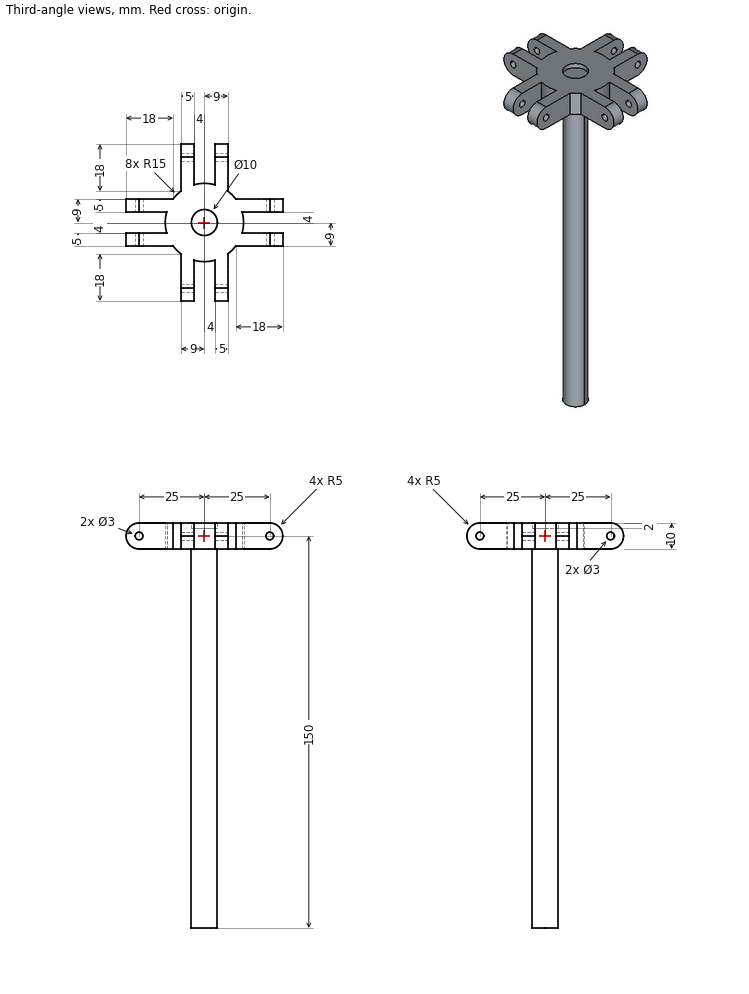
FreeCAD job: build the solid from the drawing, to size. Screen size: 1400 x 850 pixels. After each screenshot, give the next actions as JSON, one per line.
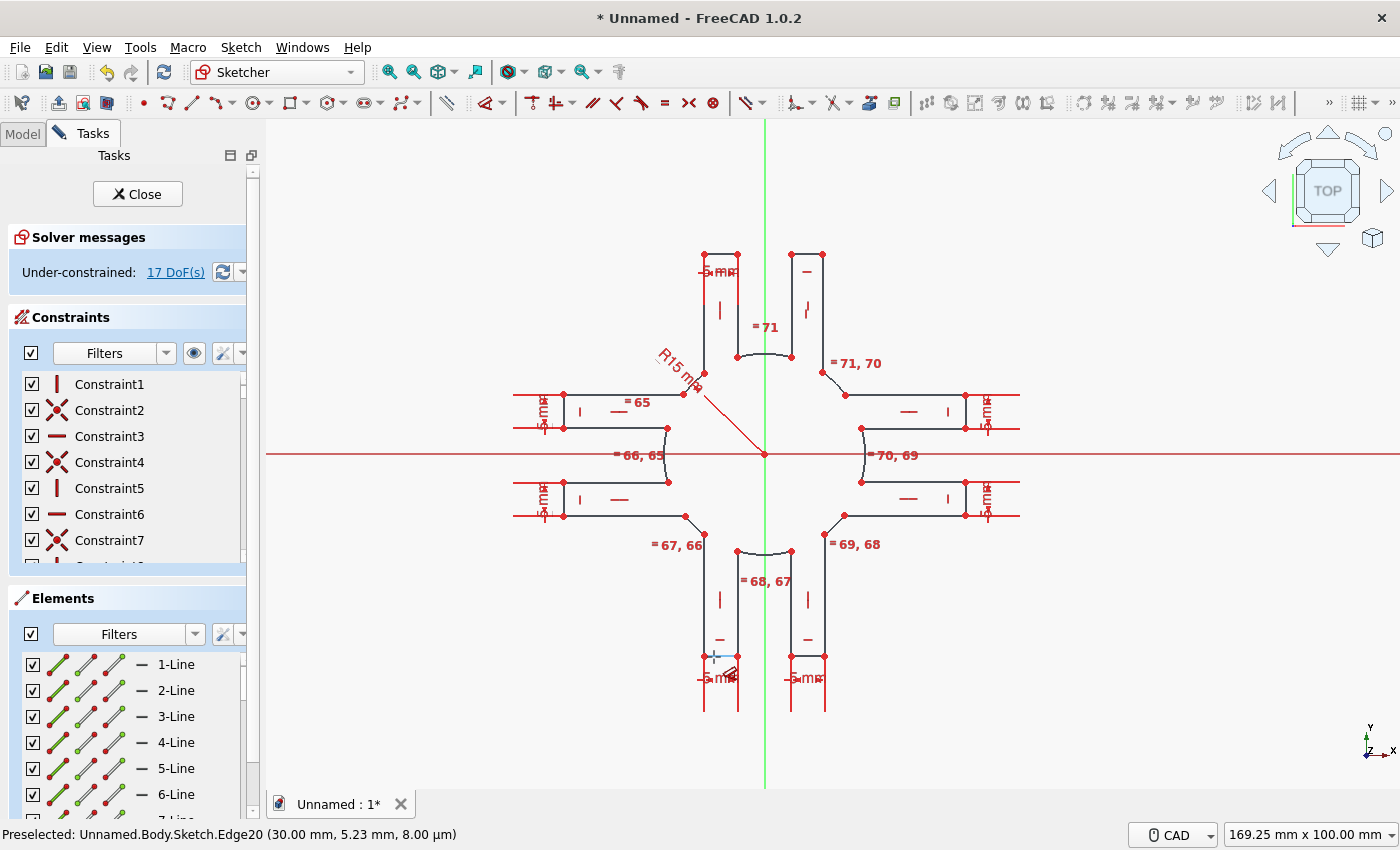
{"action": "scroll", "coordinate": [813, 254], "scroll_direction": "up", "scroll_amount": 2}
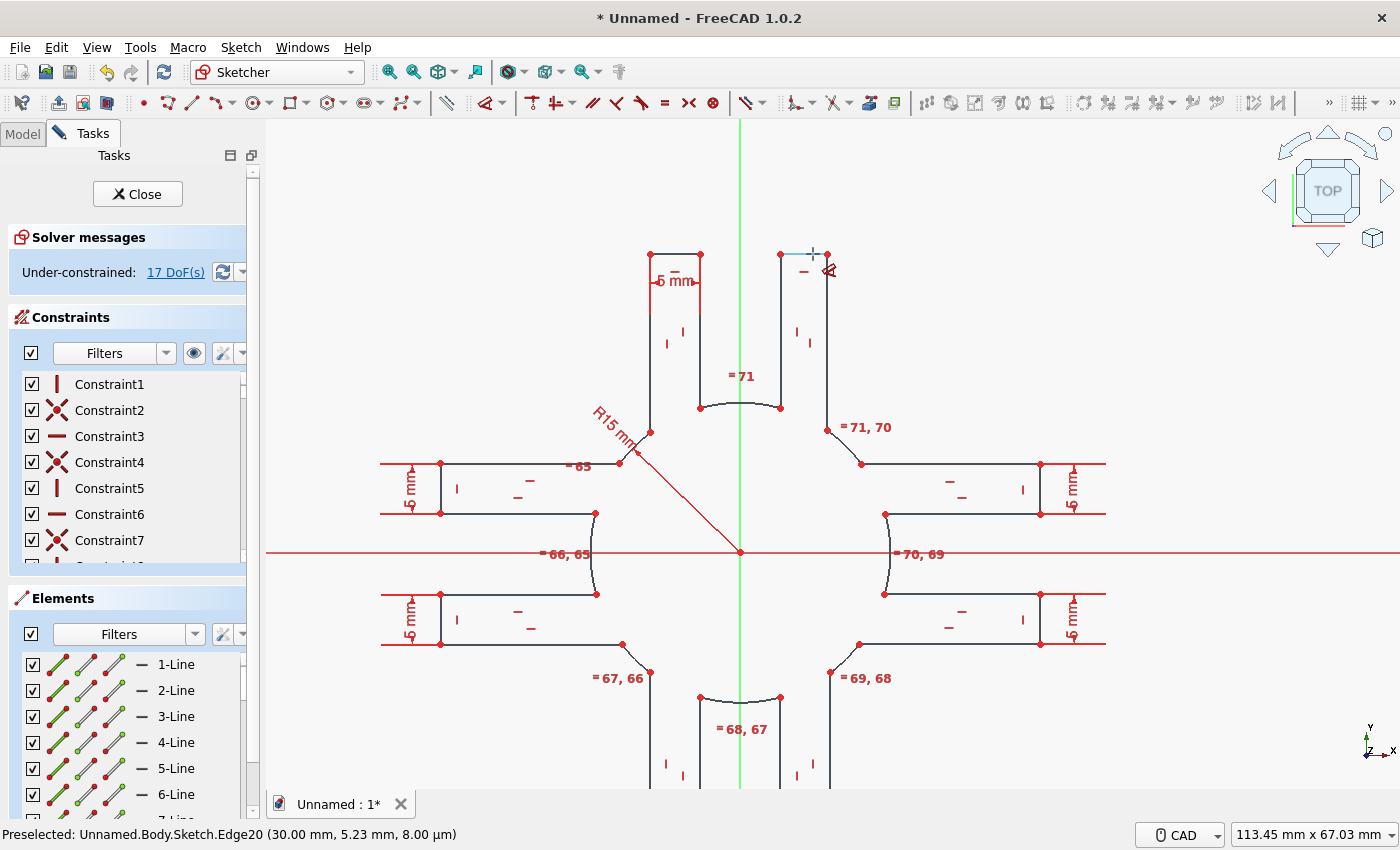
{"action": "left_click", "coordinate": [813, 254]}
{"action": "left_click", "coordinate": [804, 220]}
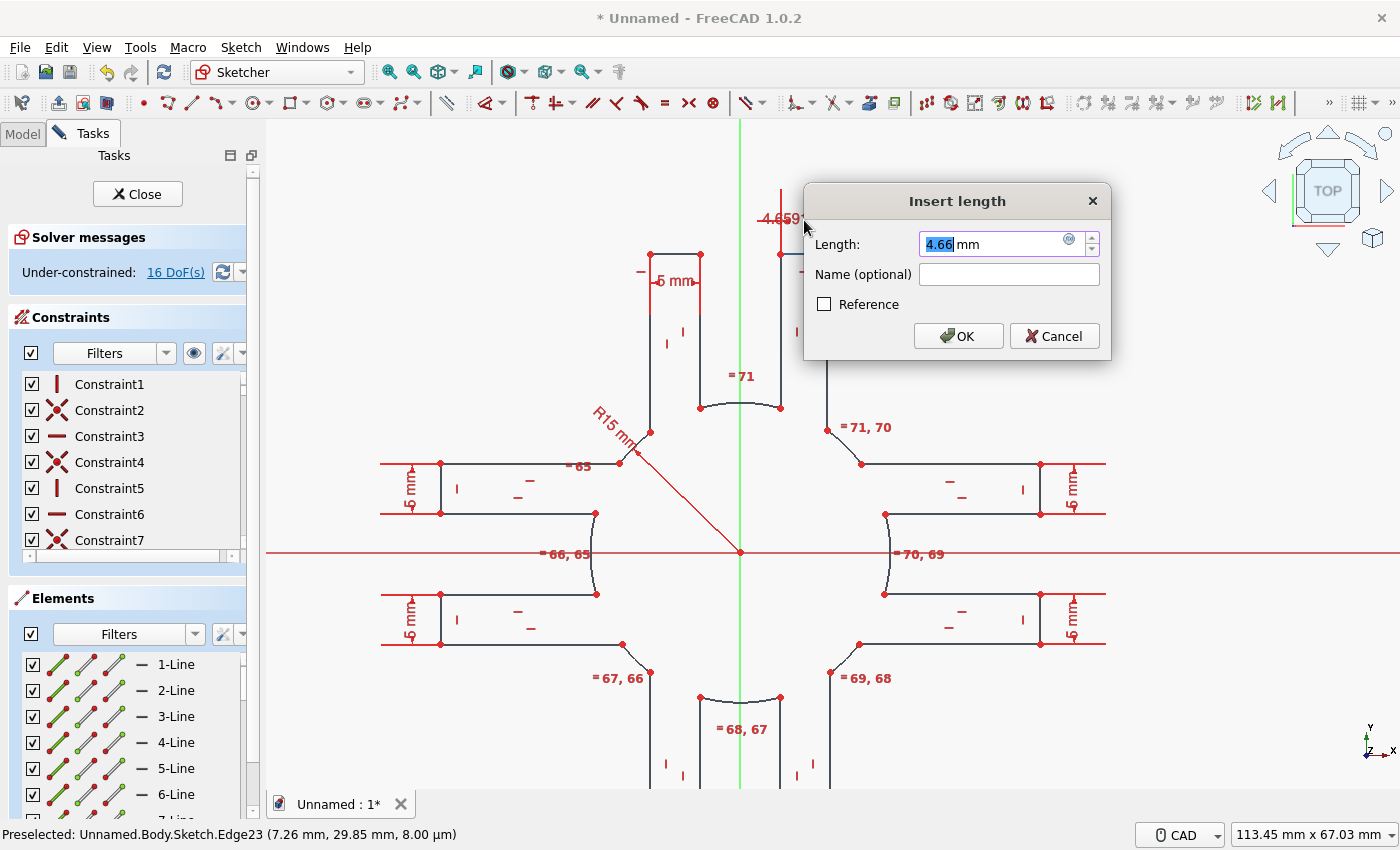
{"action": "type", "text": "5"}
{"action": "key", "text": "Return"}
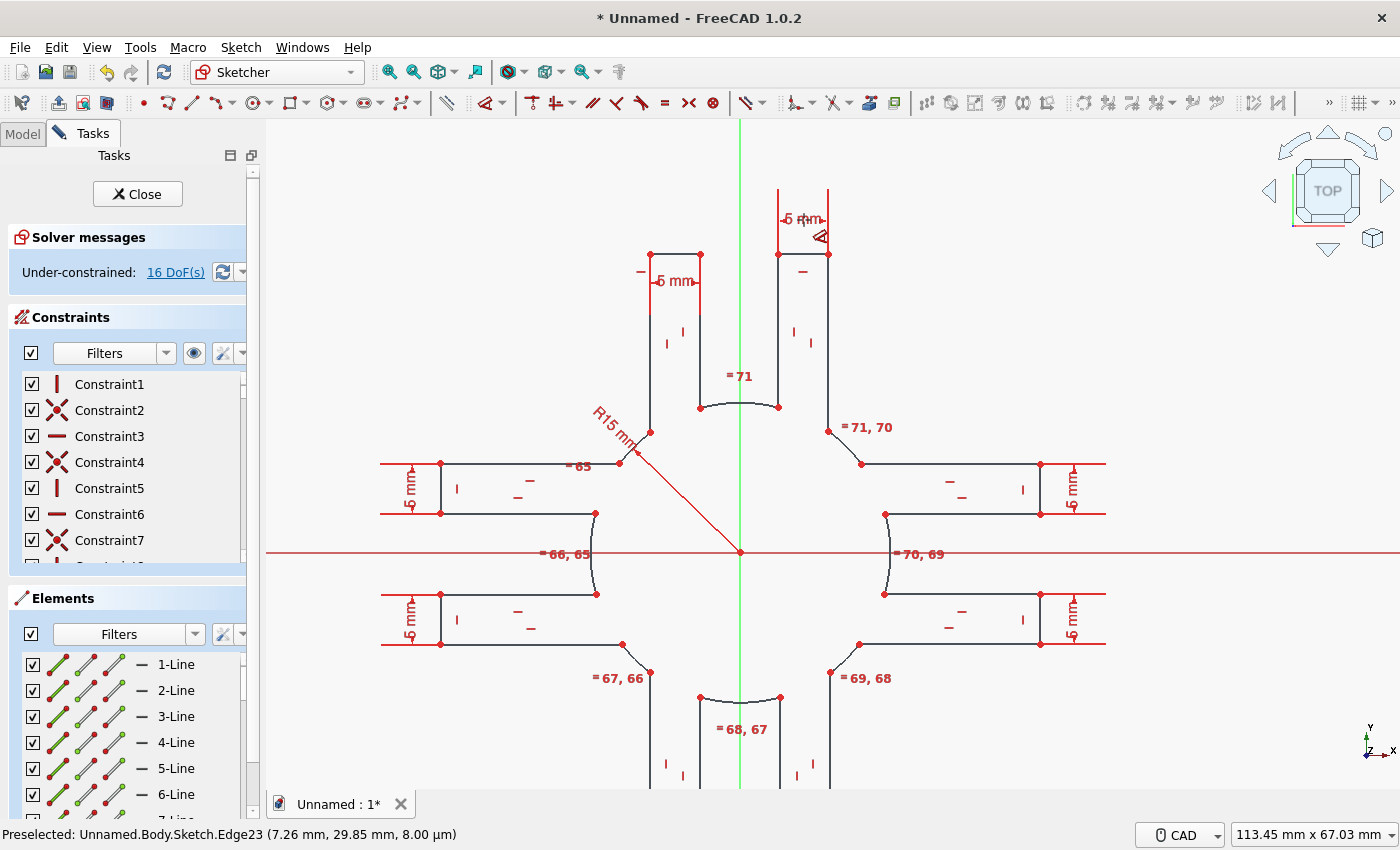
{"action": "left_click", "coordinate": [650, 308]}
{"action": "left_click", "coordinate": [616, 344]}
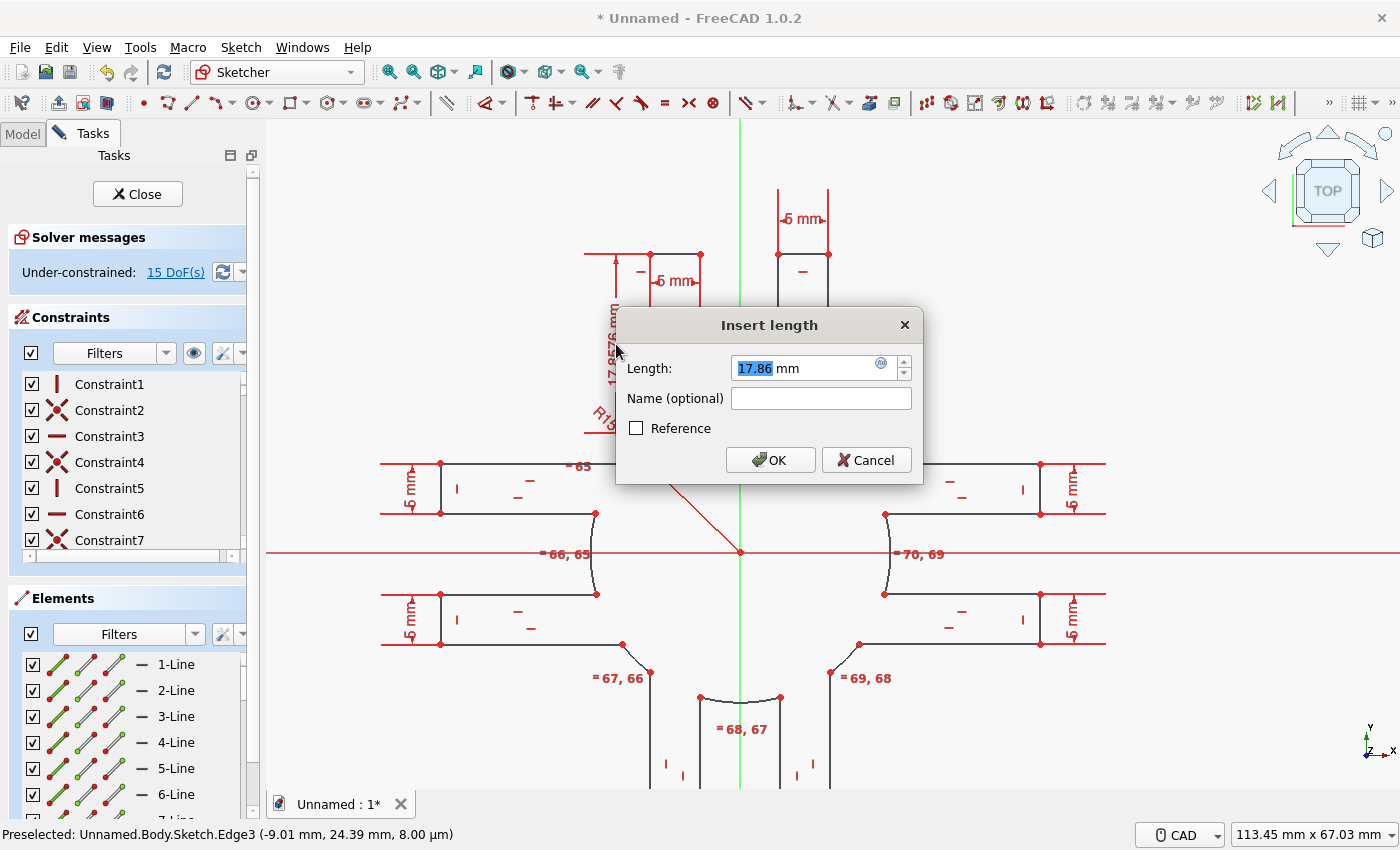
{"action": "type", "text": "18"}
{"action": "key", "text": "Return"}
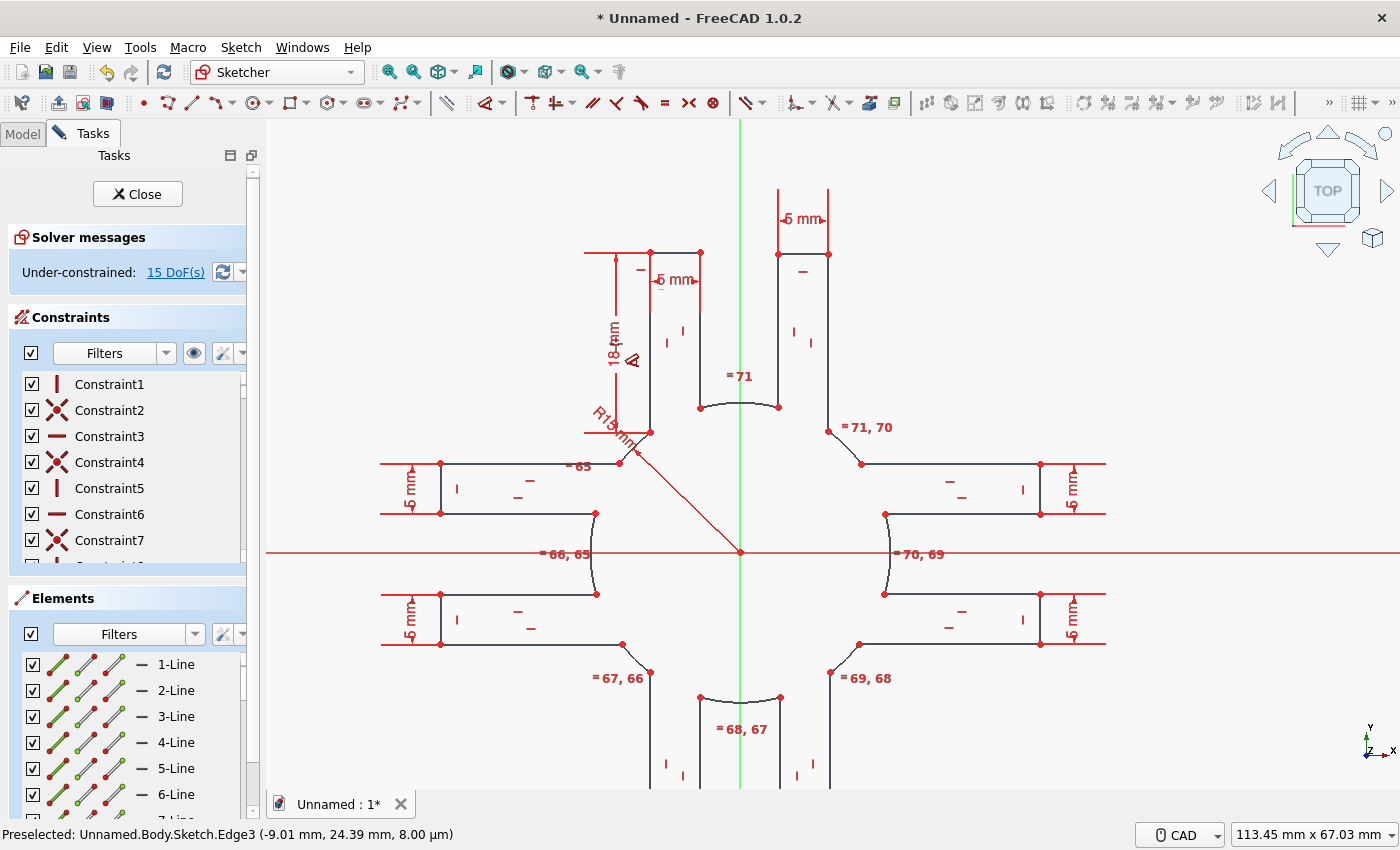
{"action": "left_click", "coordinate": [566, 464]}
{"action": "left_click", "coordinate": [530, 430]}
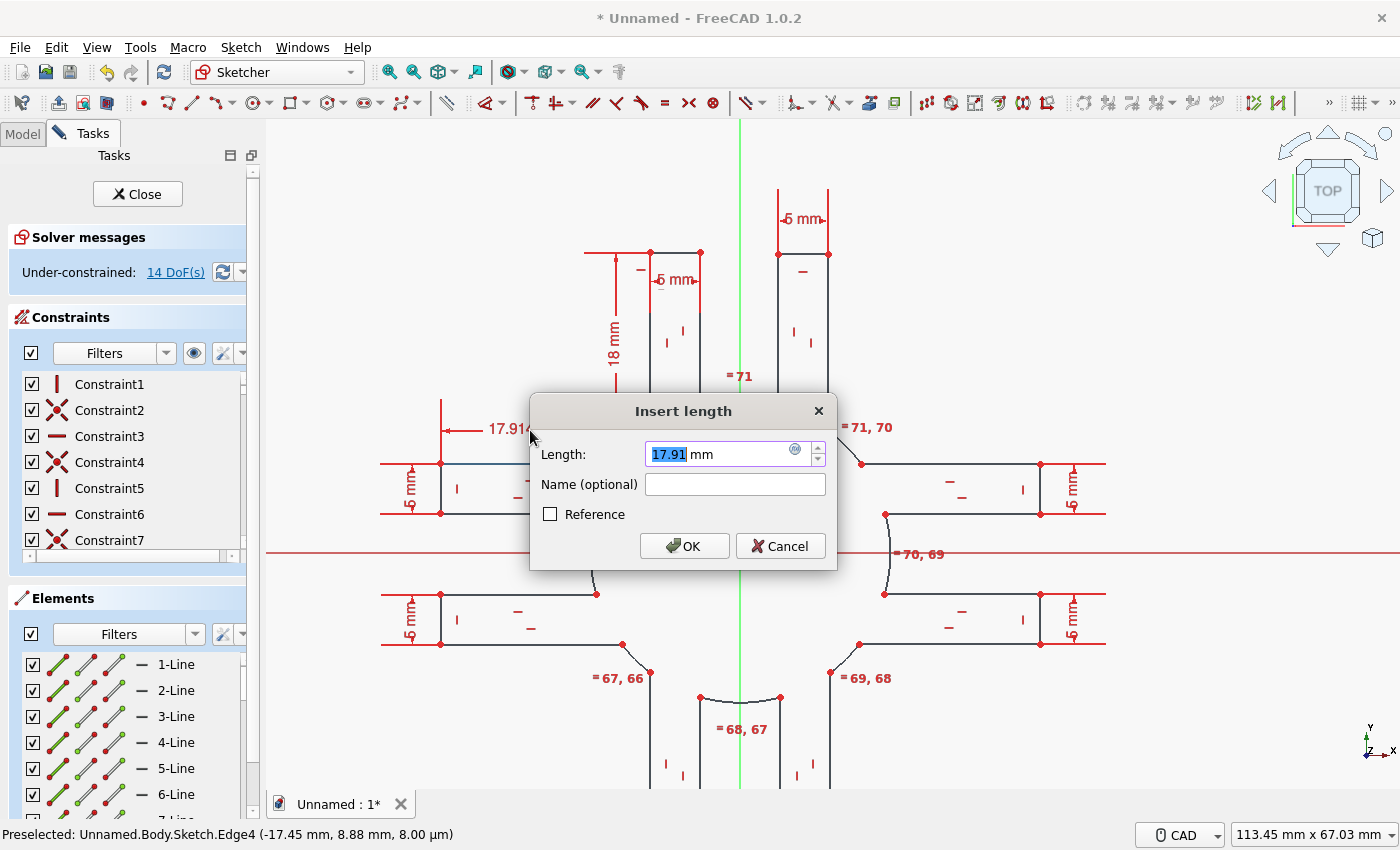
{"action": "type", "text": "18"}
{"action": "key", "text": "Return"}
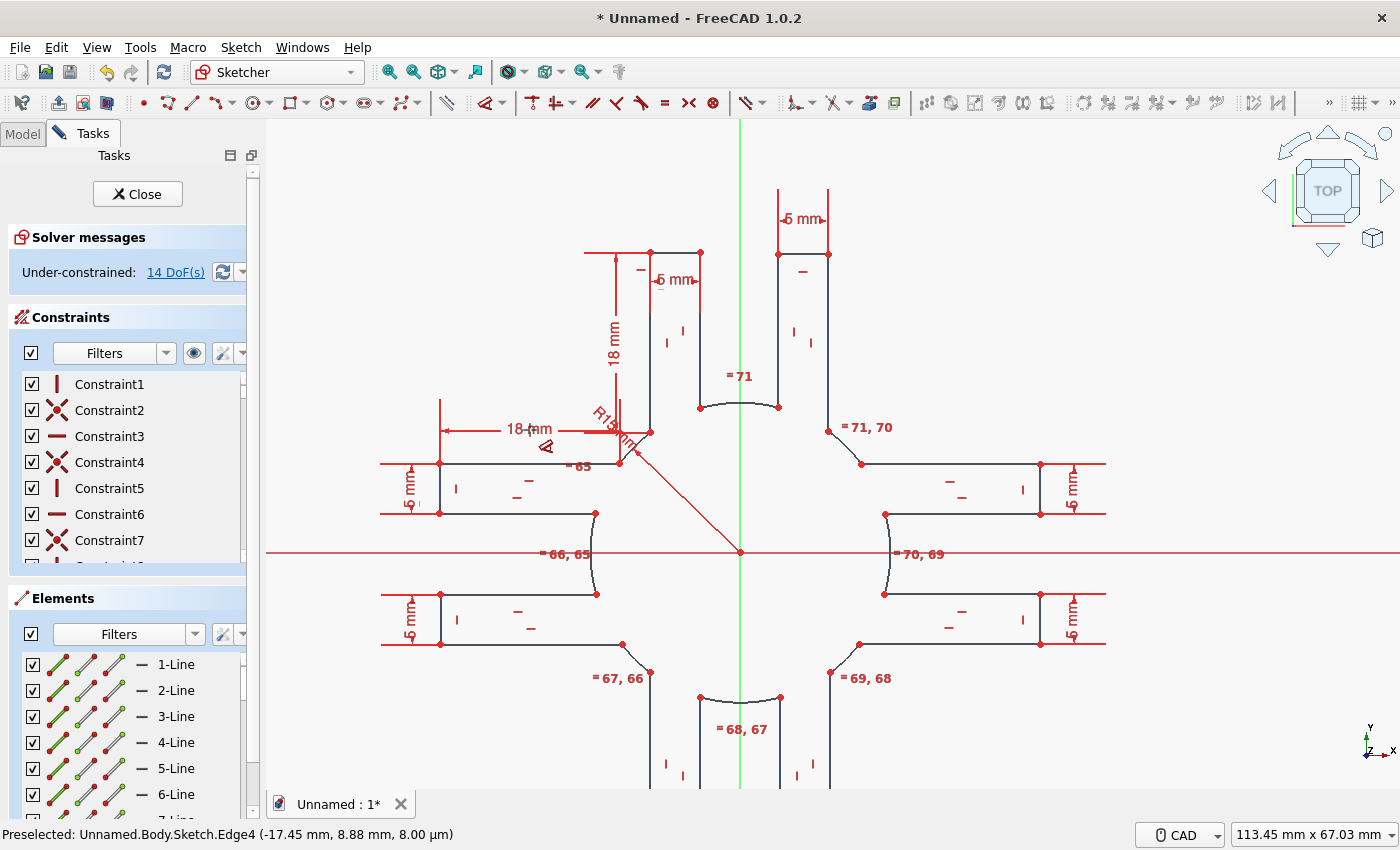
{"action": "left_click", "coordinate": [495, 645]}
{"action": "left_click", "coordinate": [531, 679]}